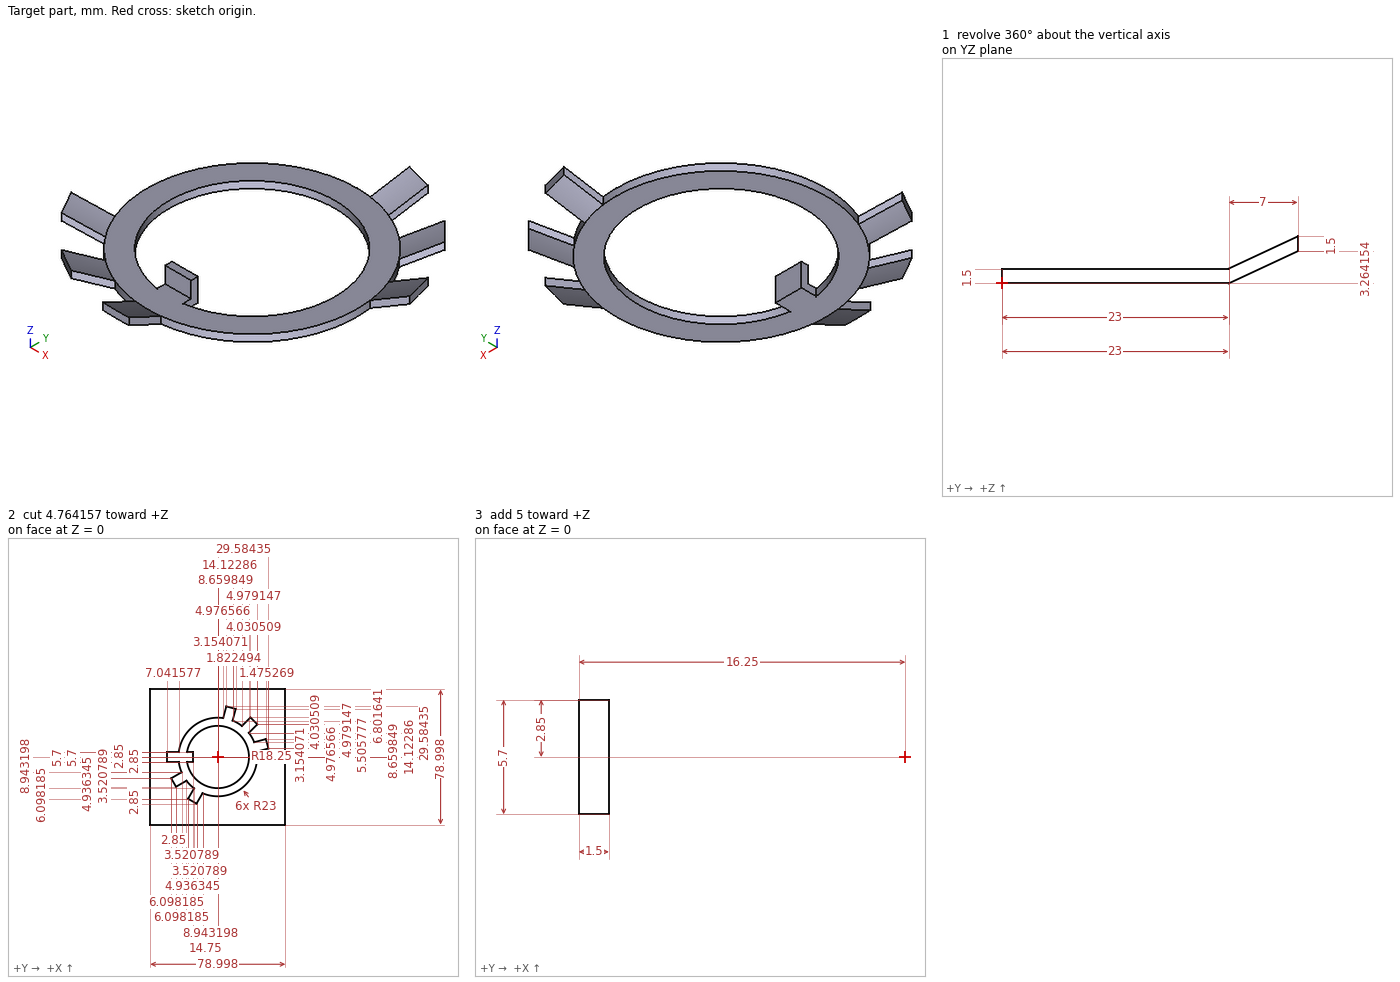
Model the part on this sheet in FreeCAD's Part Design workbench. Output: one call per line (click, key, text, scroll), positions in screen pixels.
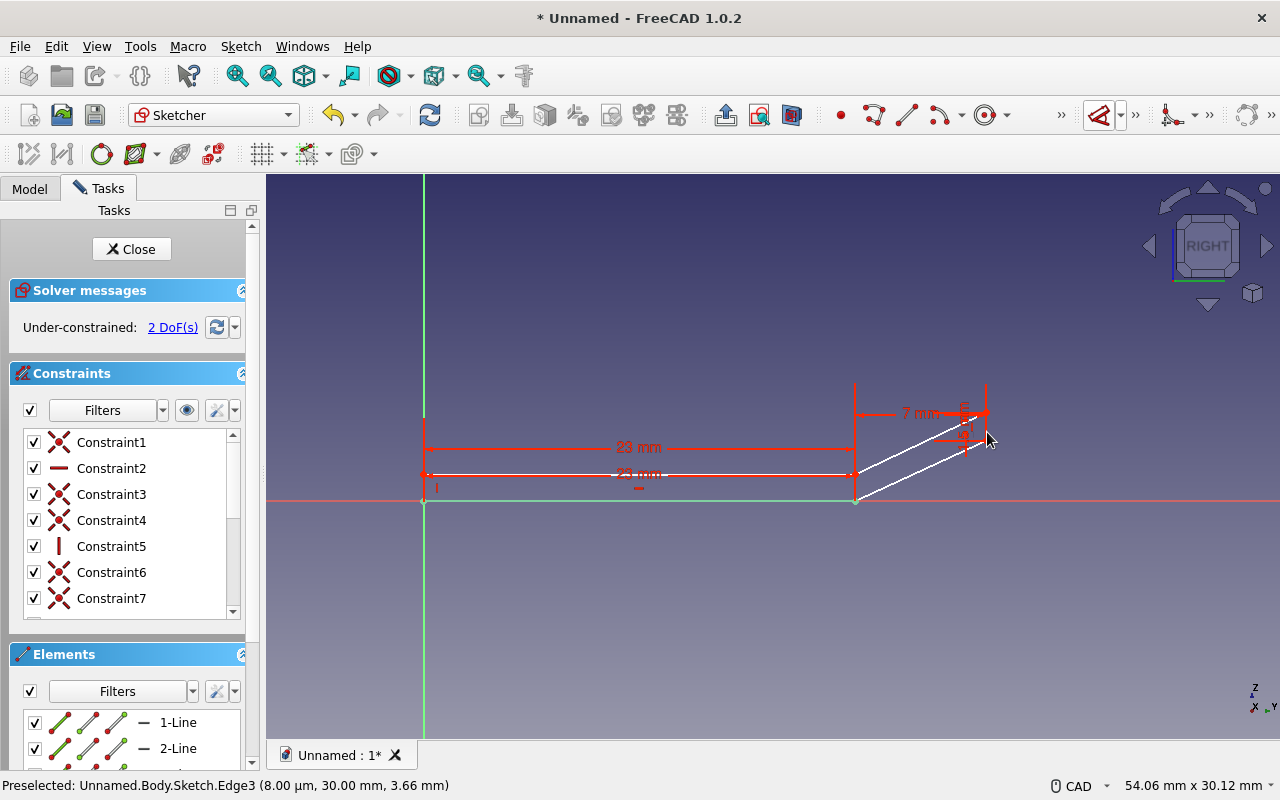
scroll(424, 483, up, 3)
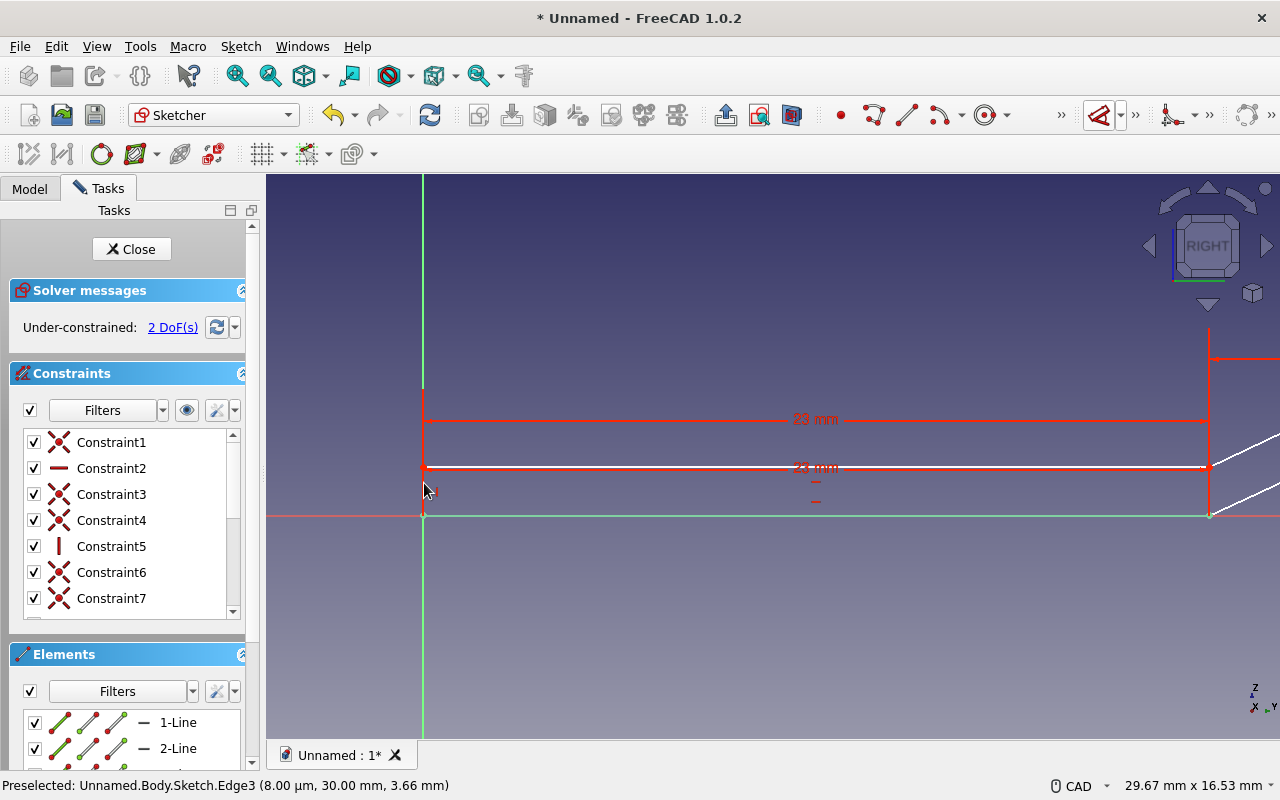
click(423, 482)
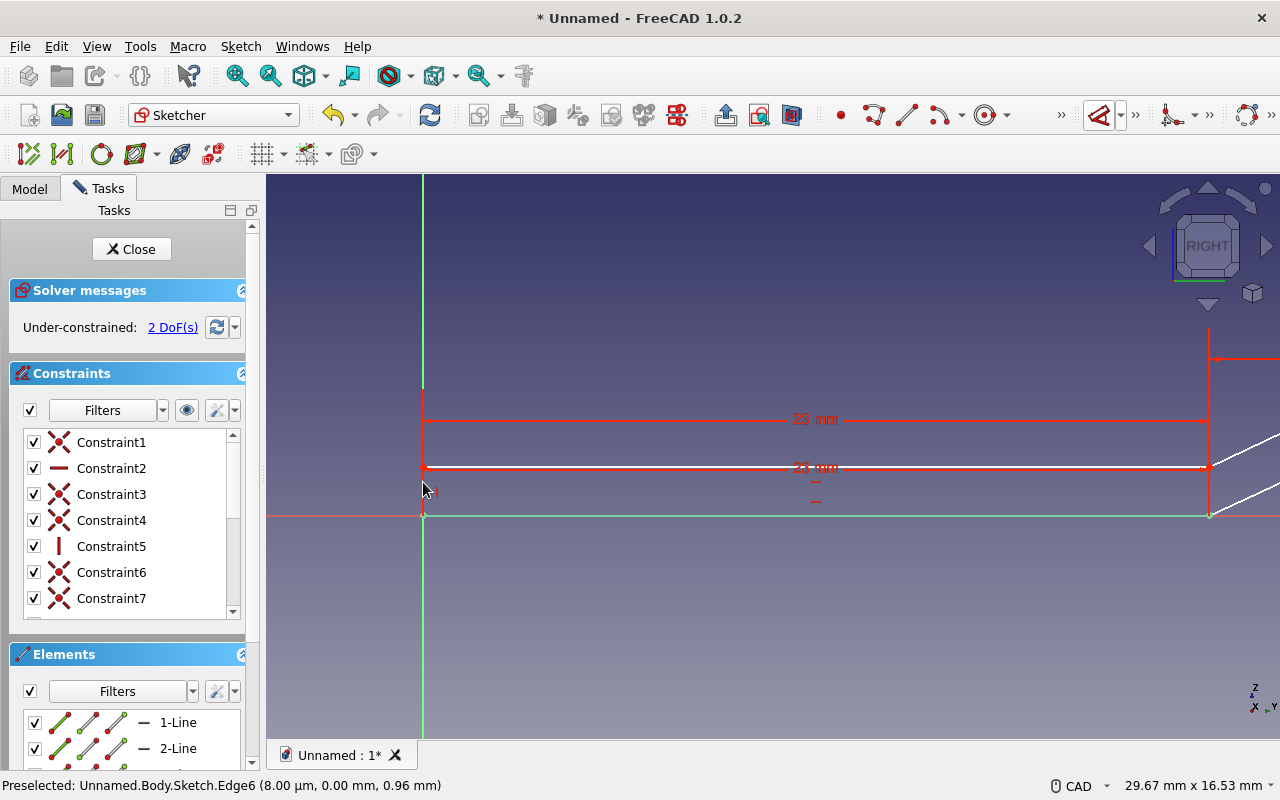
key(i)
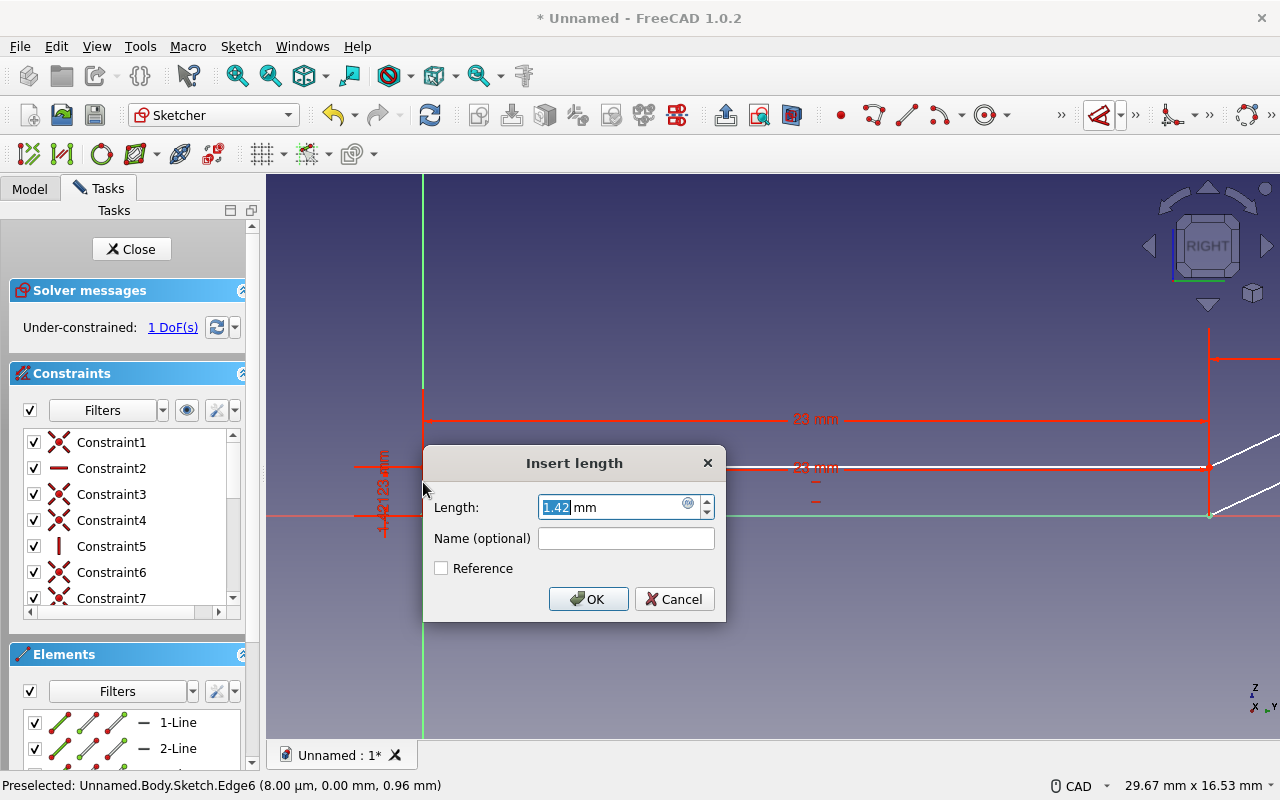
text(1.5)
key(Return)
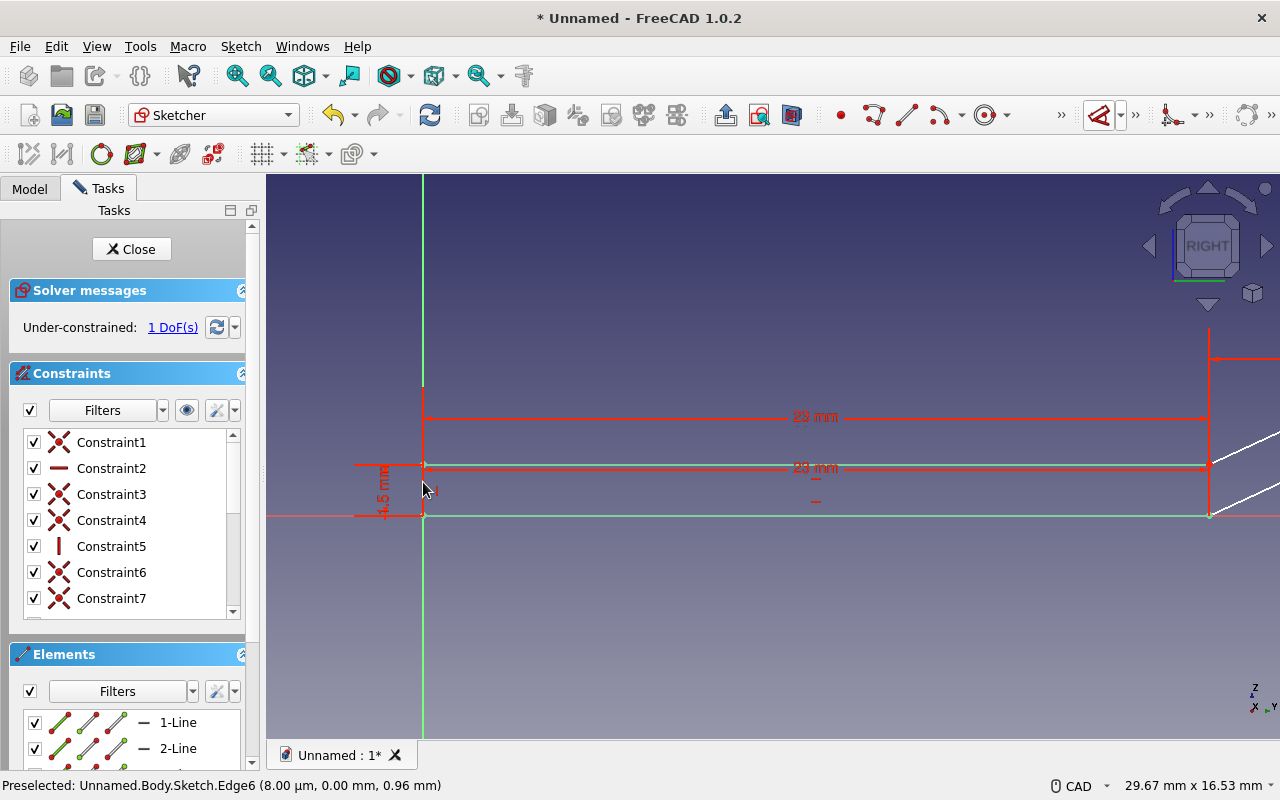
scroll(423, 483, down, 3)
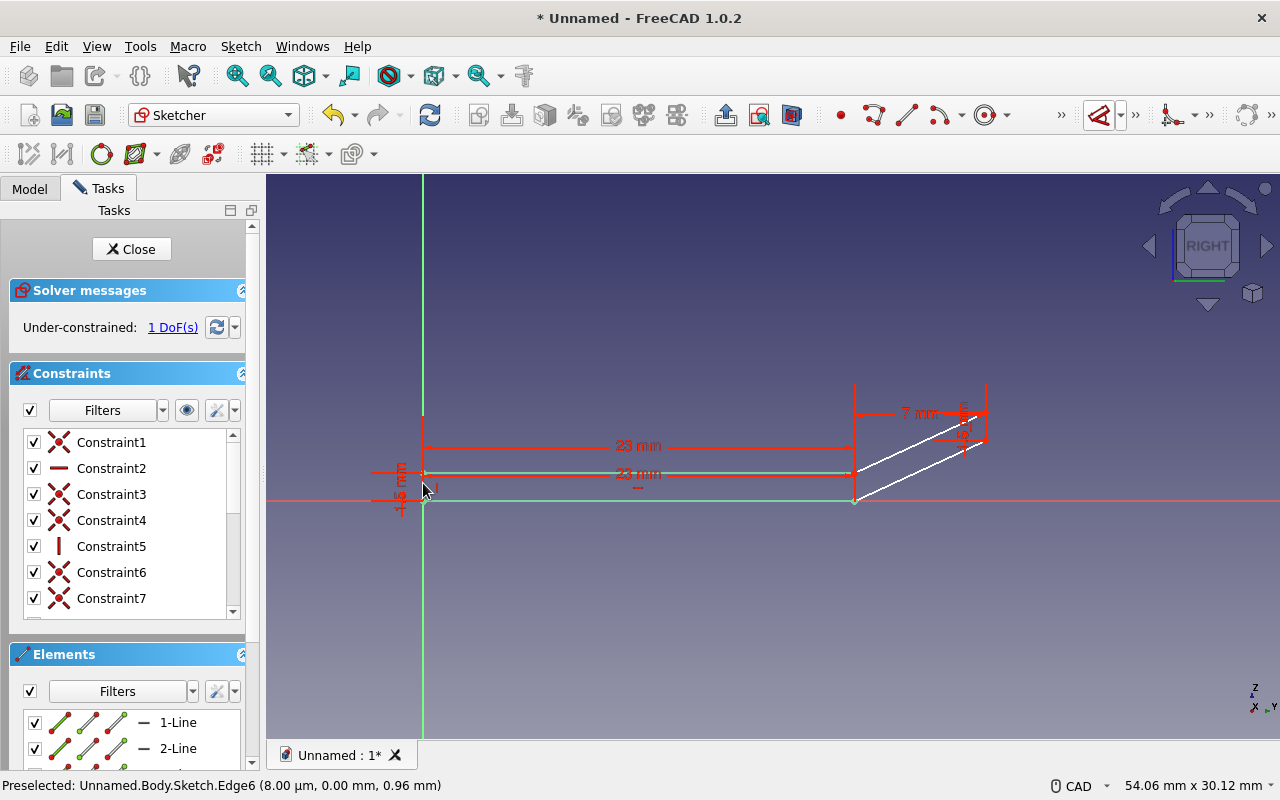
click(986, 441)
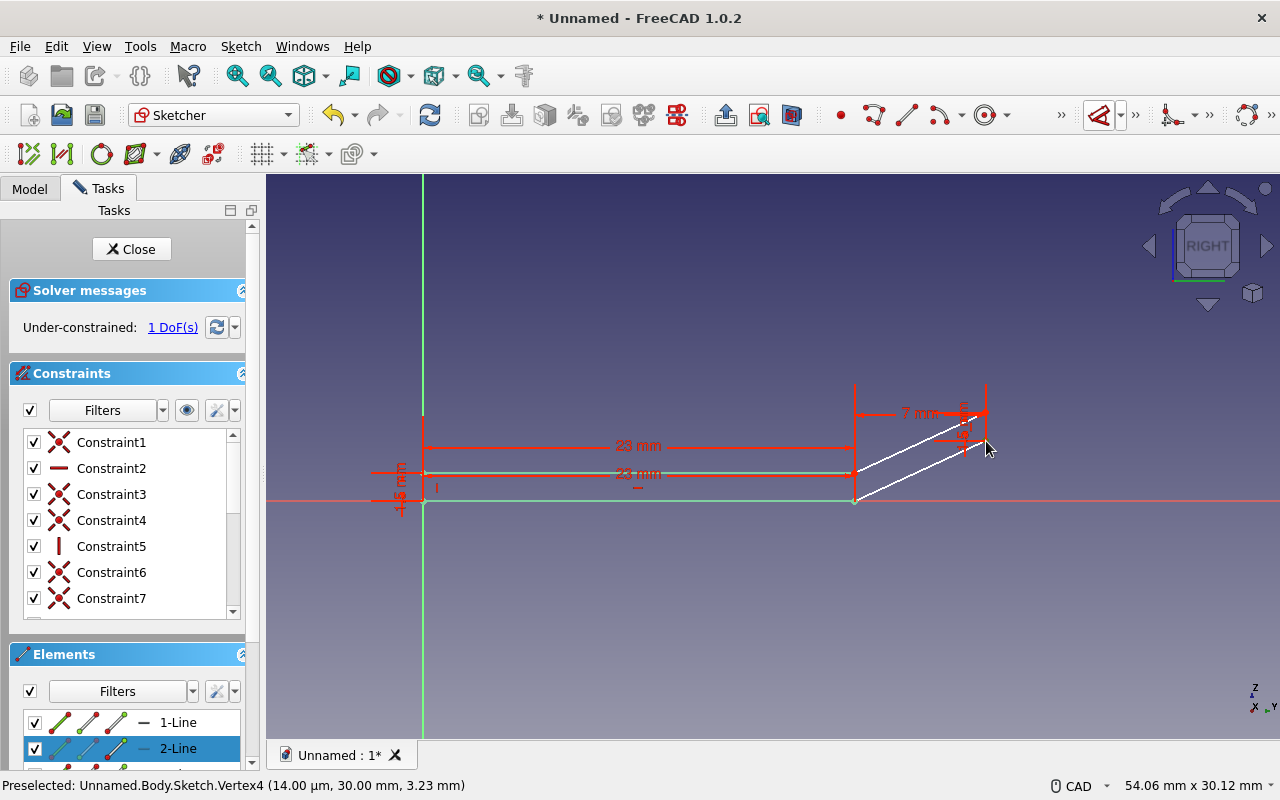
key(i)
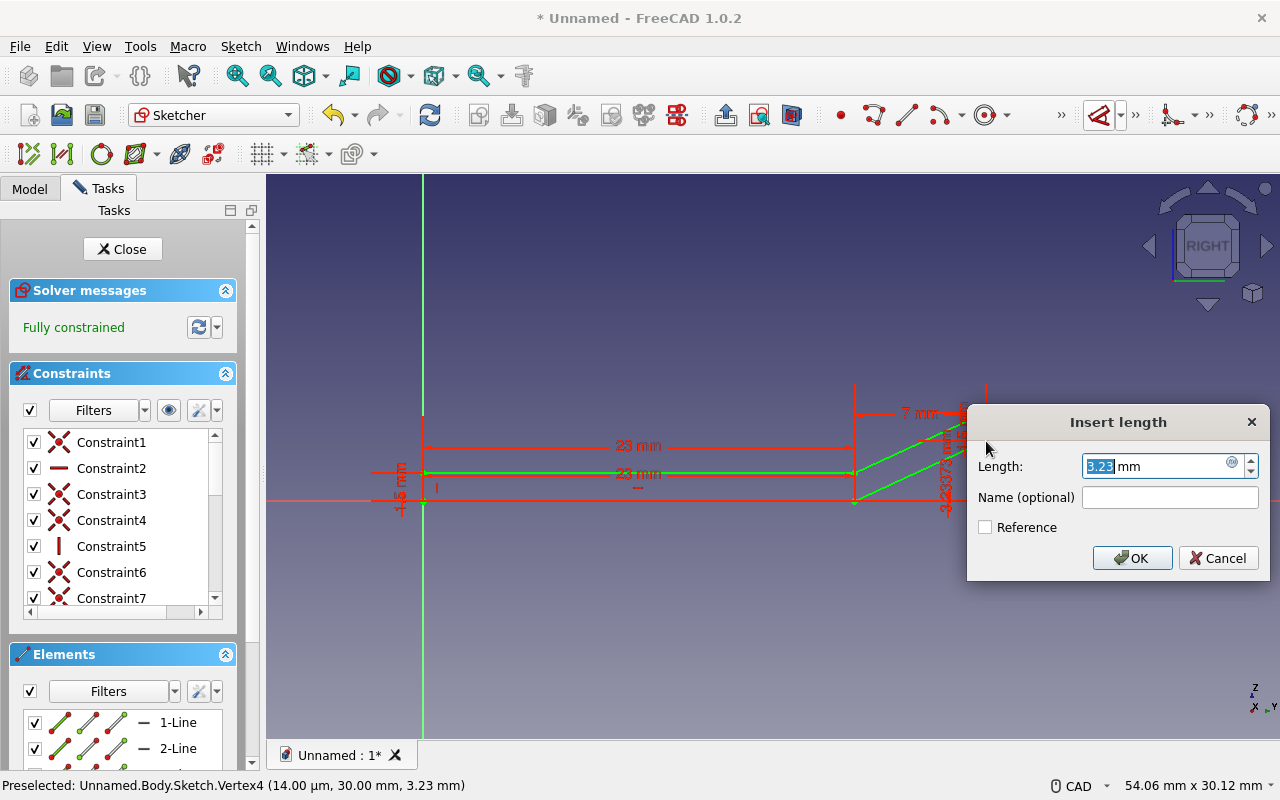
text(3.264154)
key(Return)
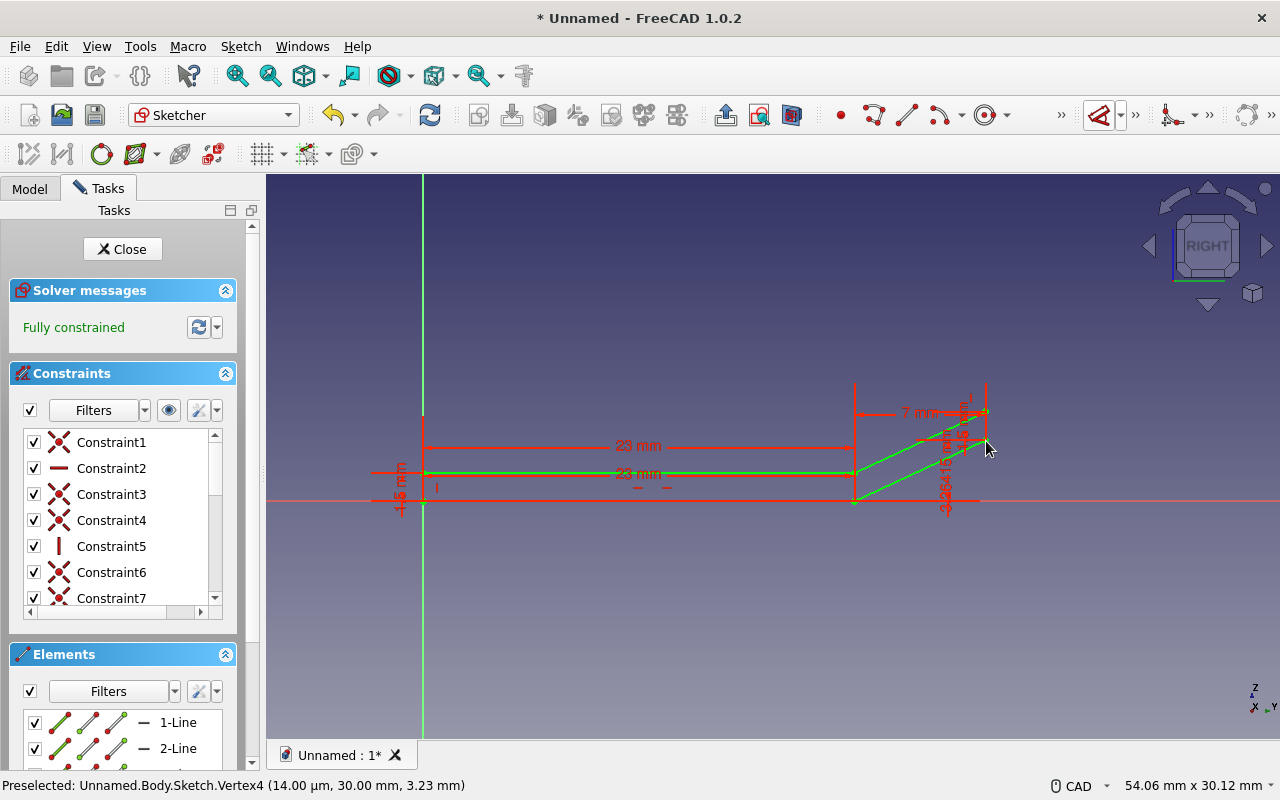
click(123, 249)